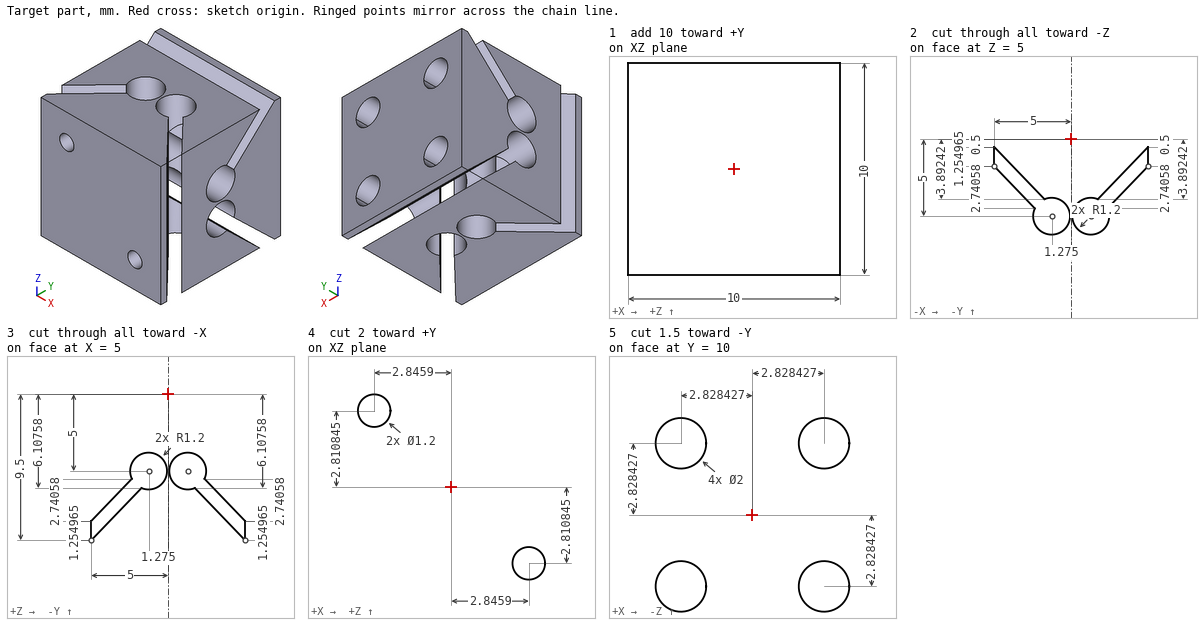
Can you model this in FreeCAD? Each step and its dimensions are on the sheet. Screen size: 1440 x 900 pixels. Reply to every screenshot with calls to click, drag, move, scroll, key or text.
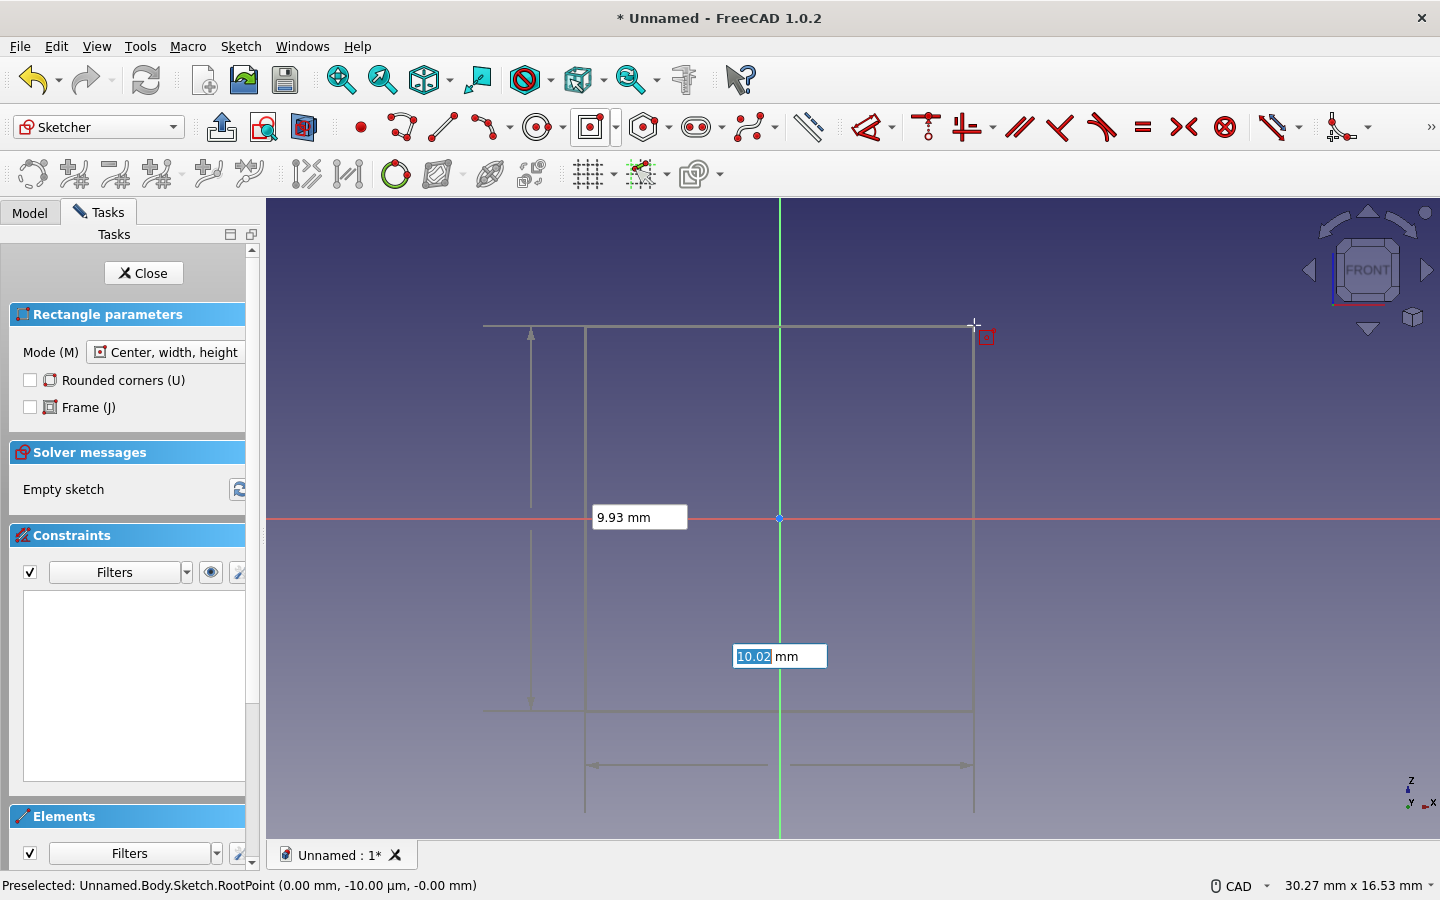
text(10)
key(Tab)
text(10)
key(Return)
key(Escape)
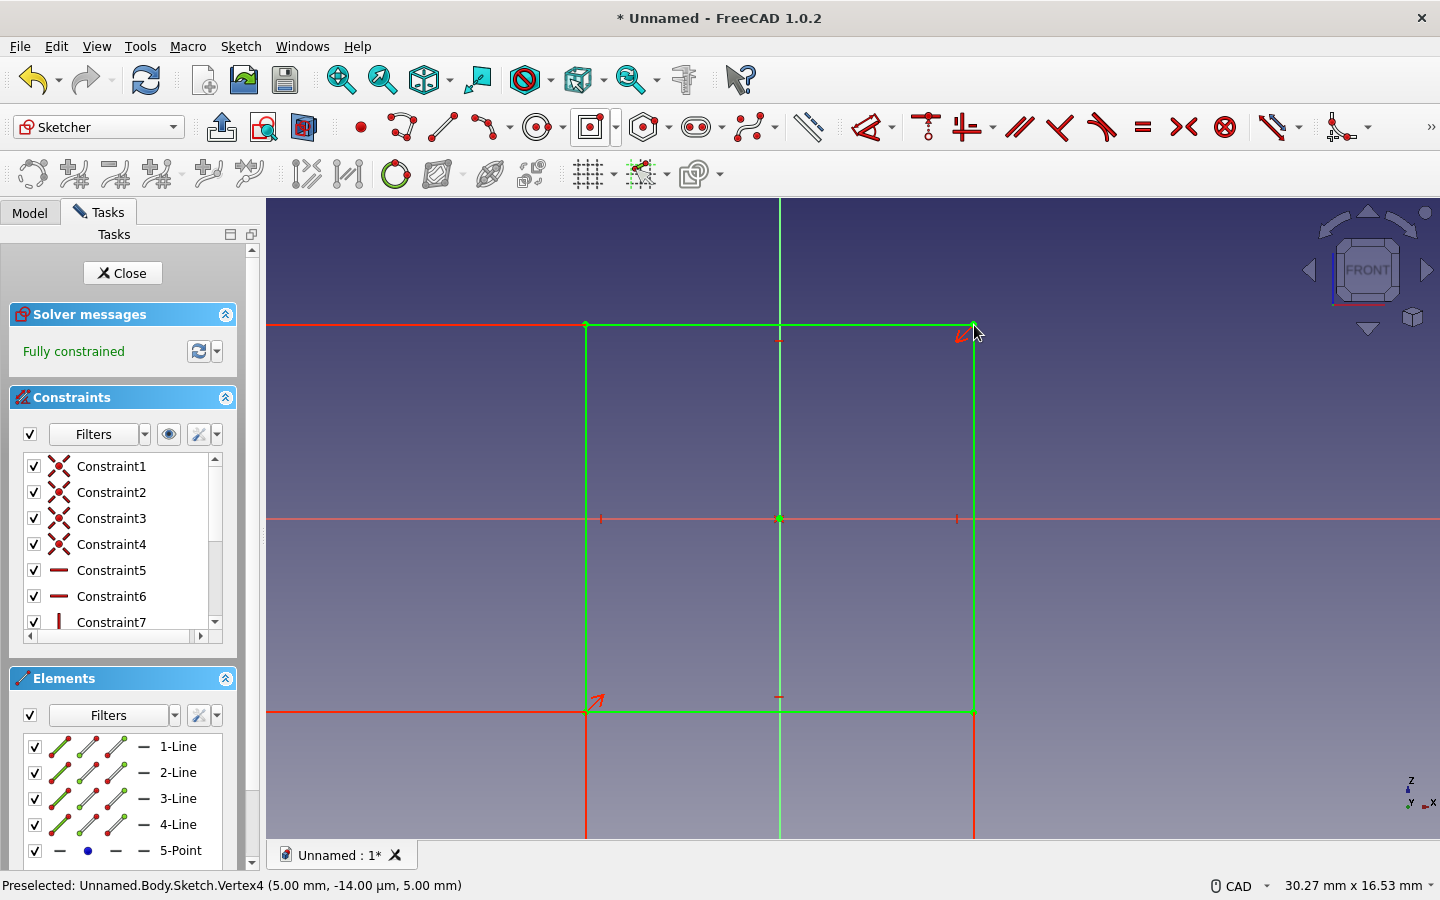
click(123, 273)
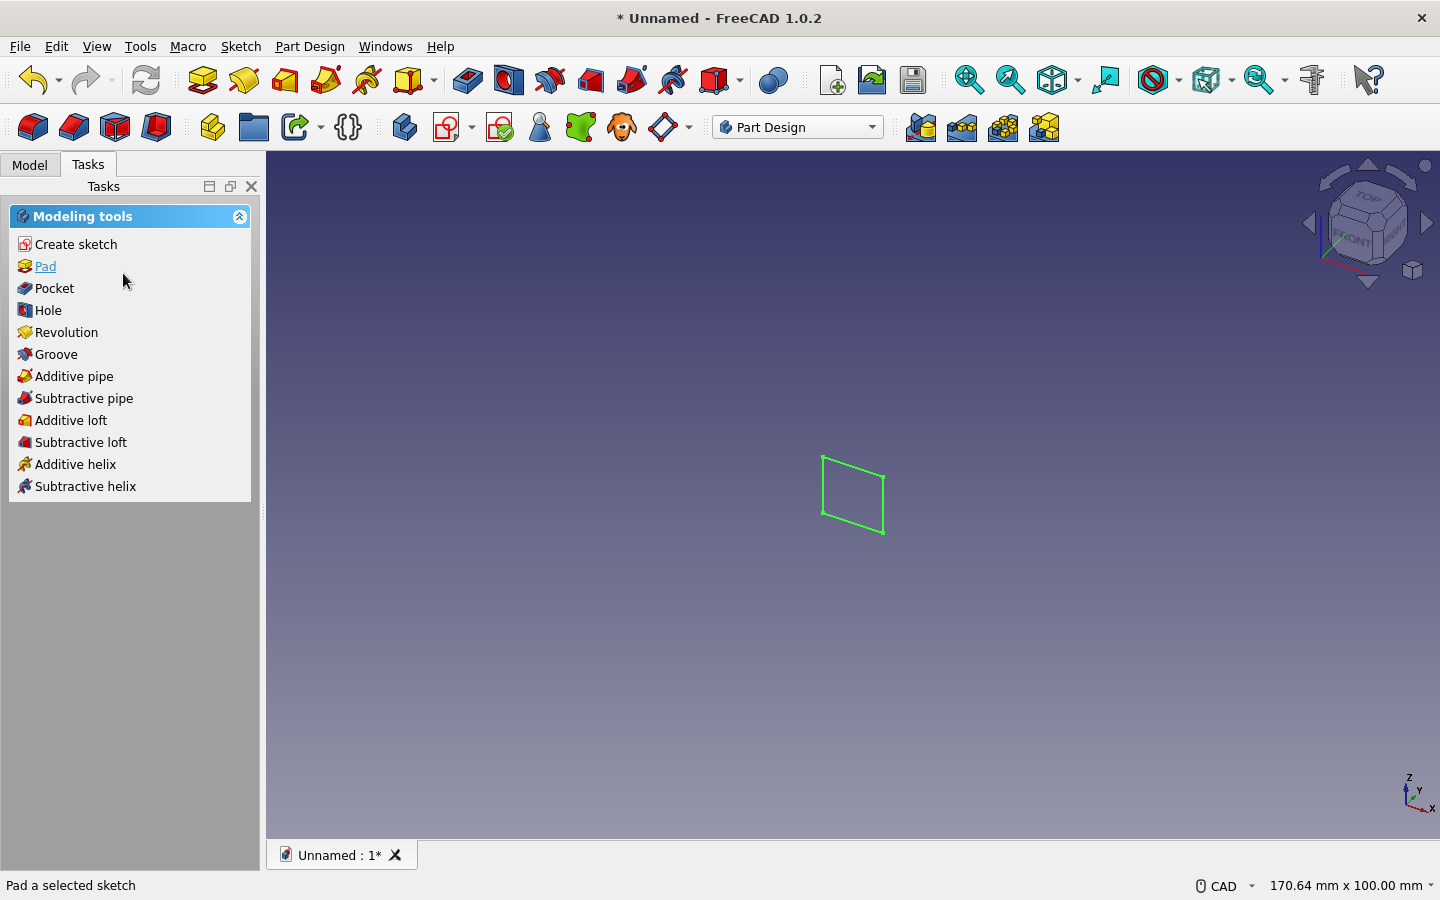
click(203, 80)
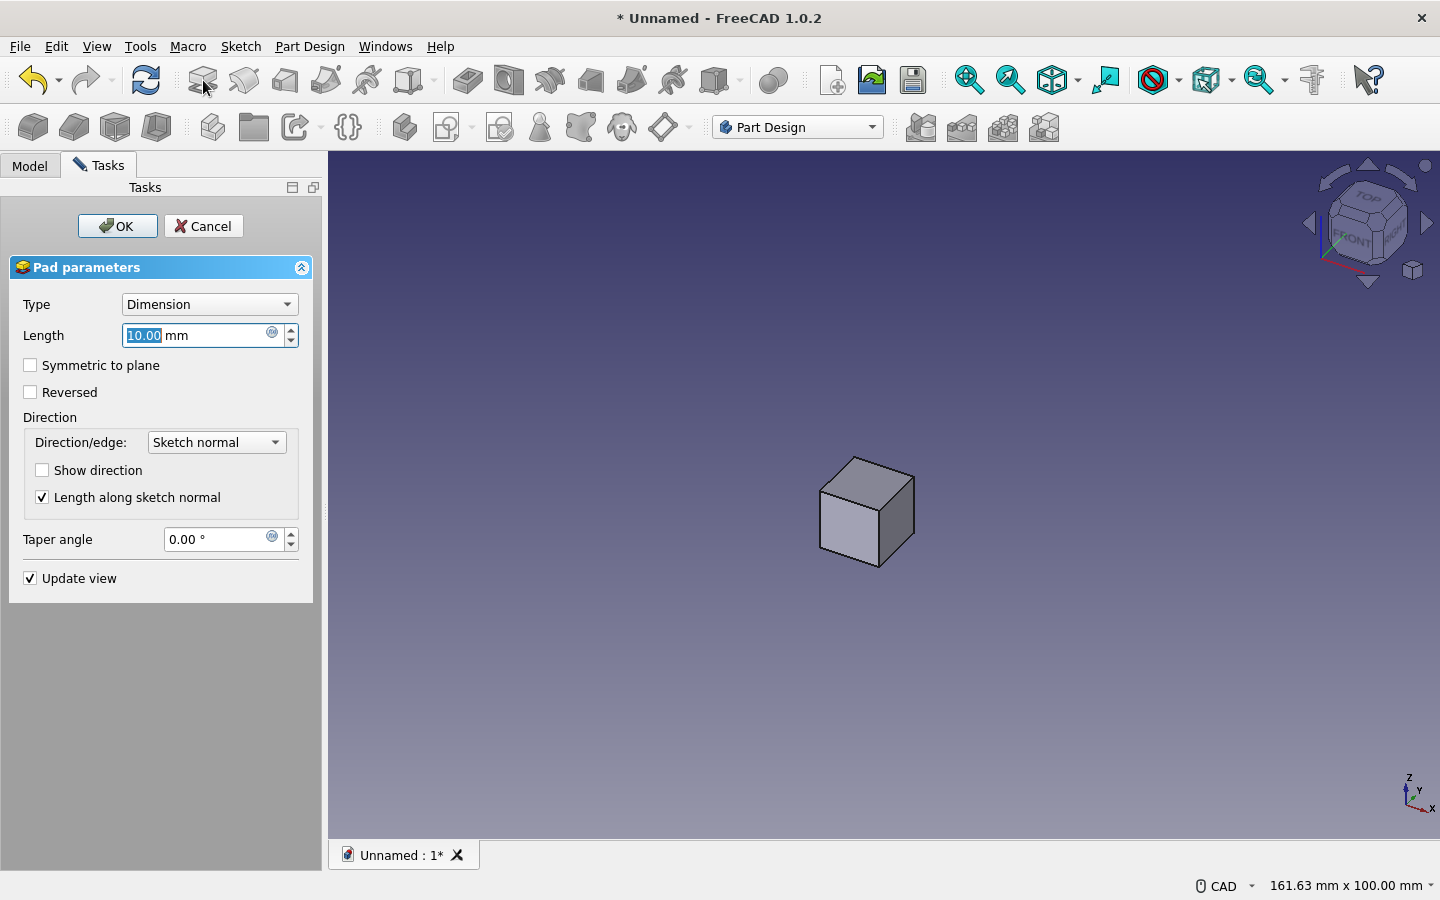
text(10)
key(Tab)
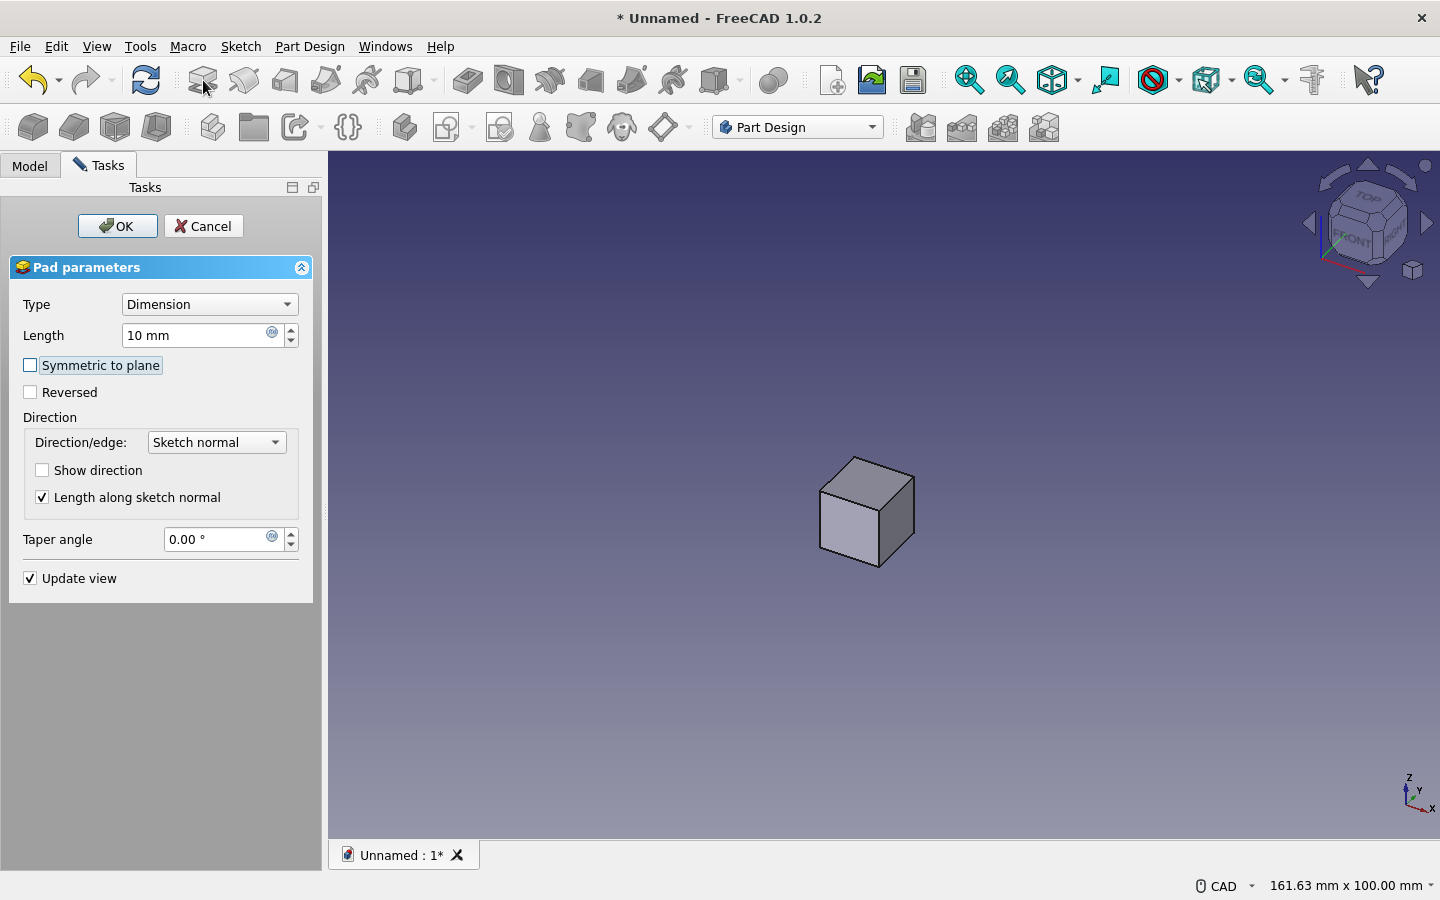
click(31, 392)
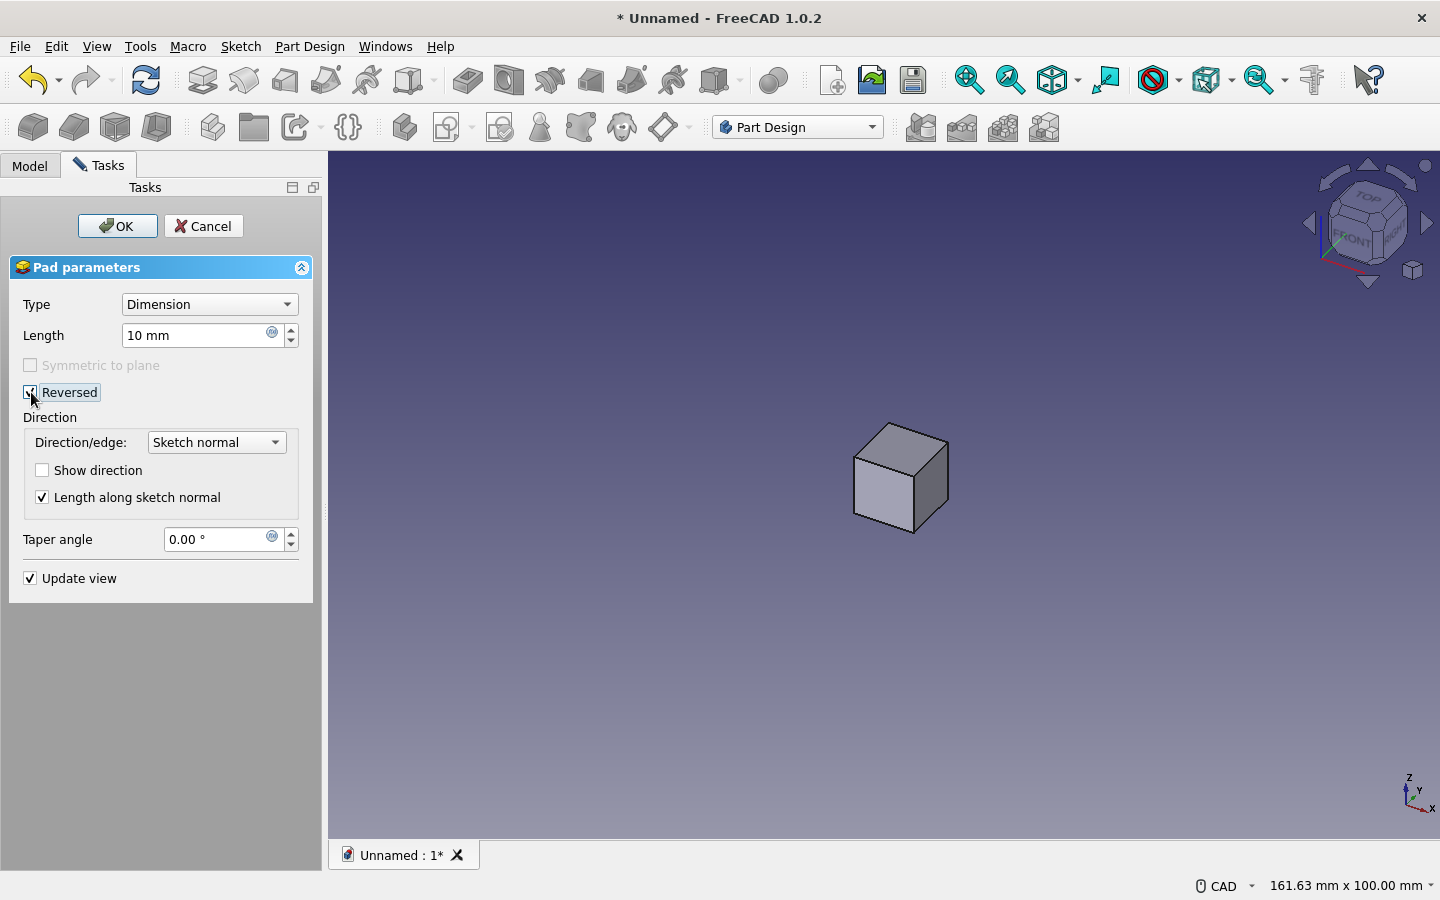
click(118, 226)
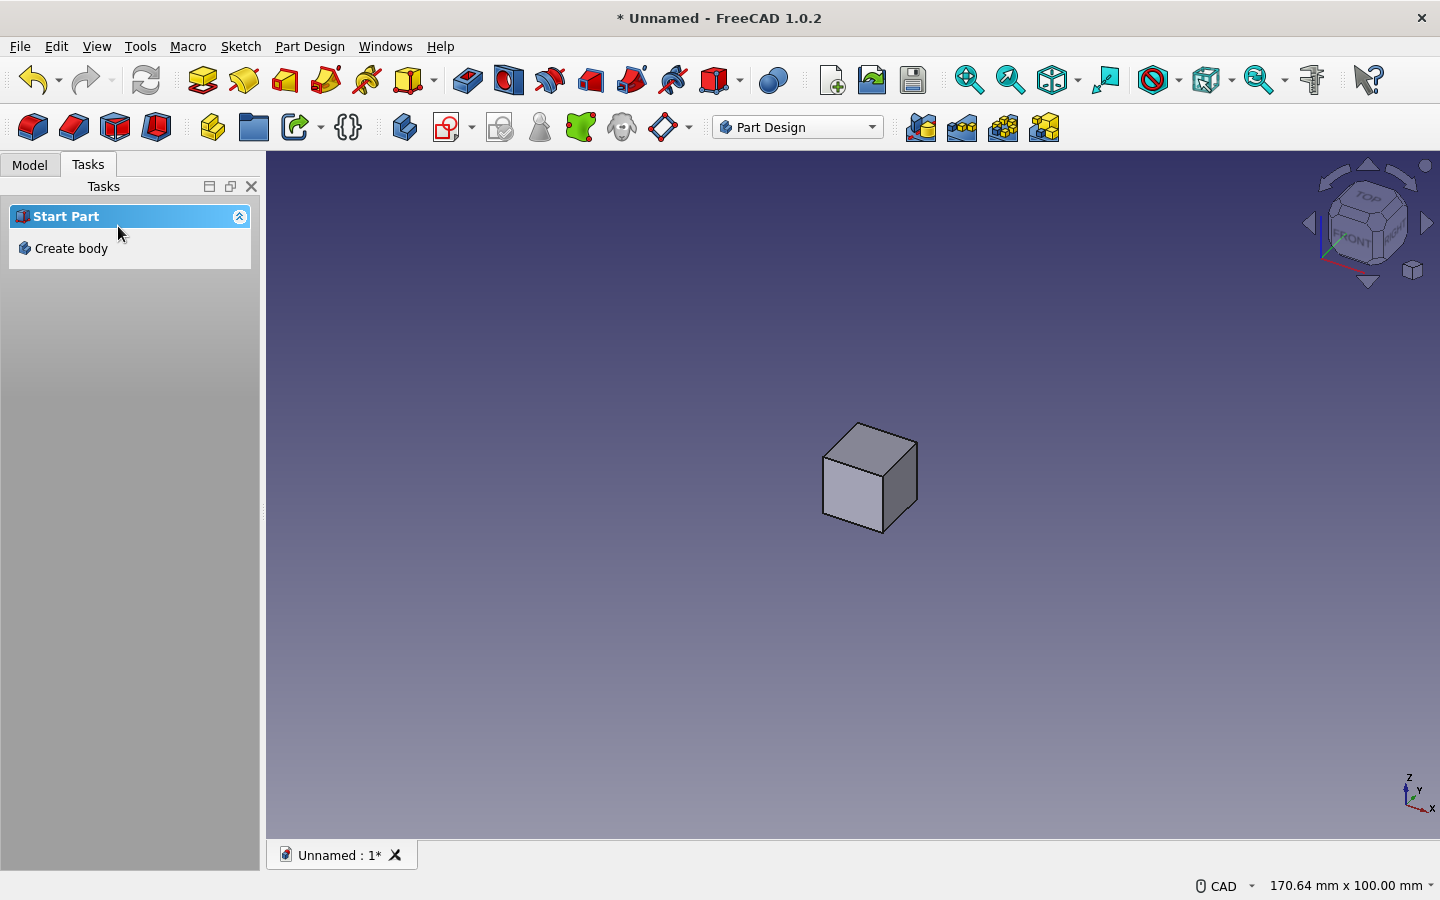
click(970, 80)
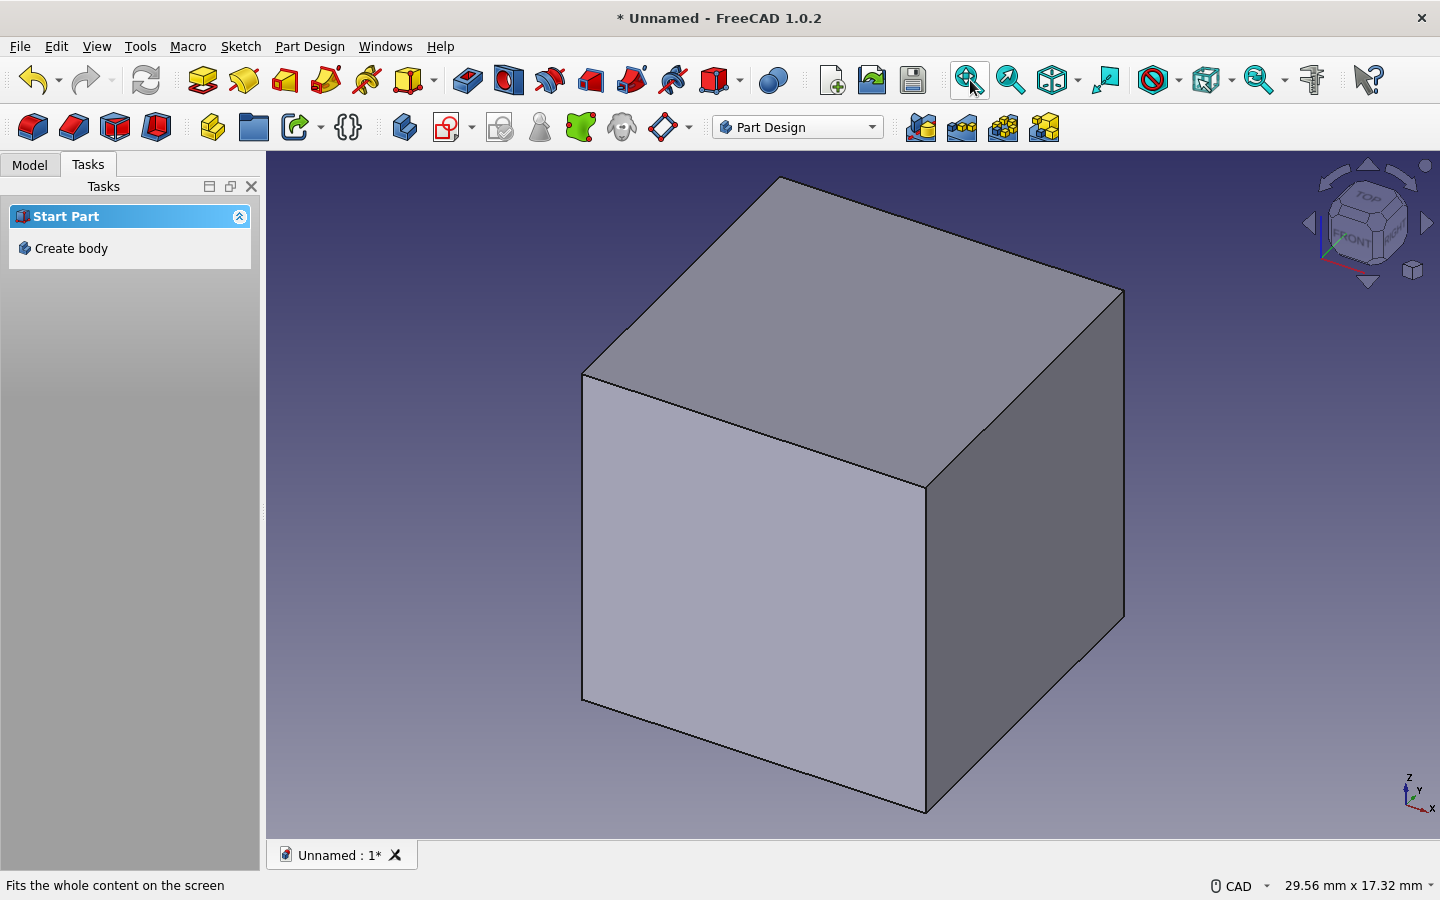
click(853, 331)